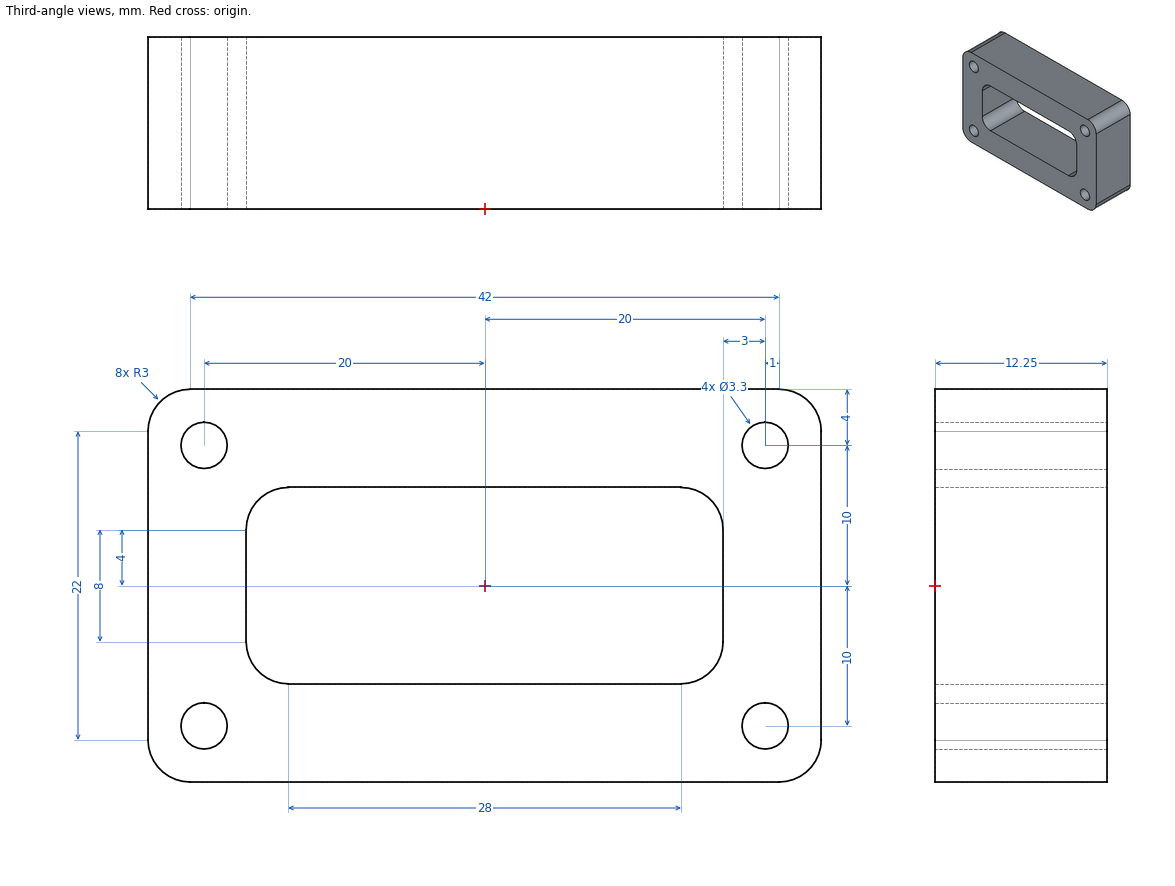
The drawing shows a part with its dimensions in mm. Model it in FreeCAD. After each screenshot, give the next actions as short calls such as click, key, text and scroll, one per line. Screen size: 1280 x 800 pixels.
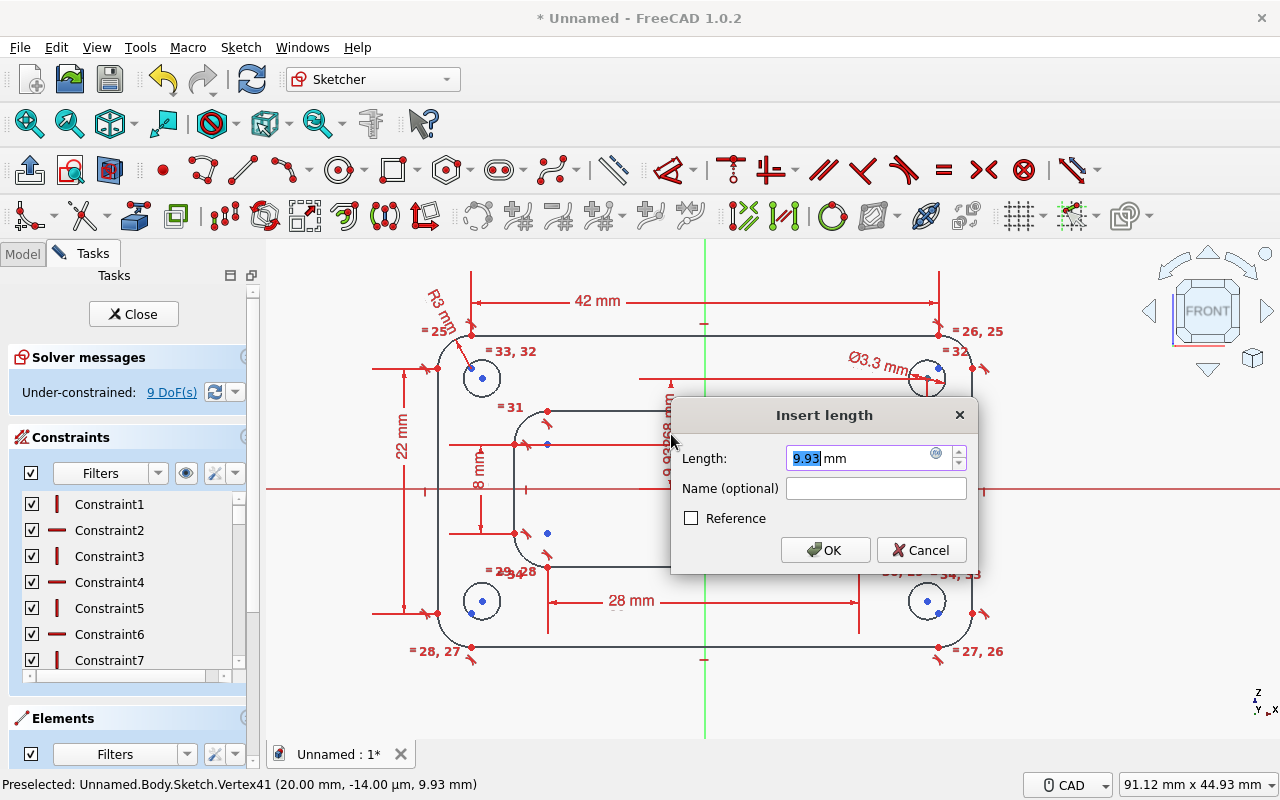
text(10)
key(Return)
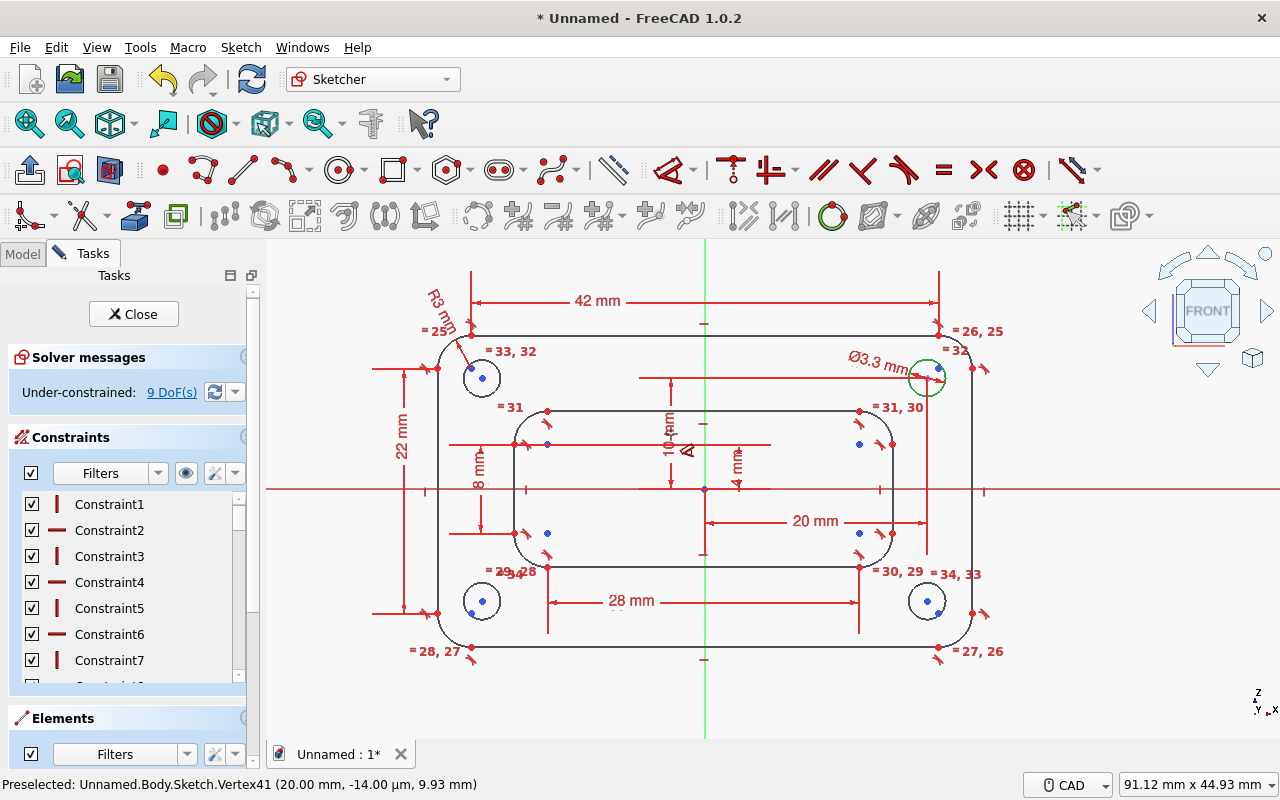
click(482, 378)
click(593, 523)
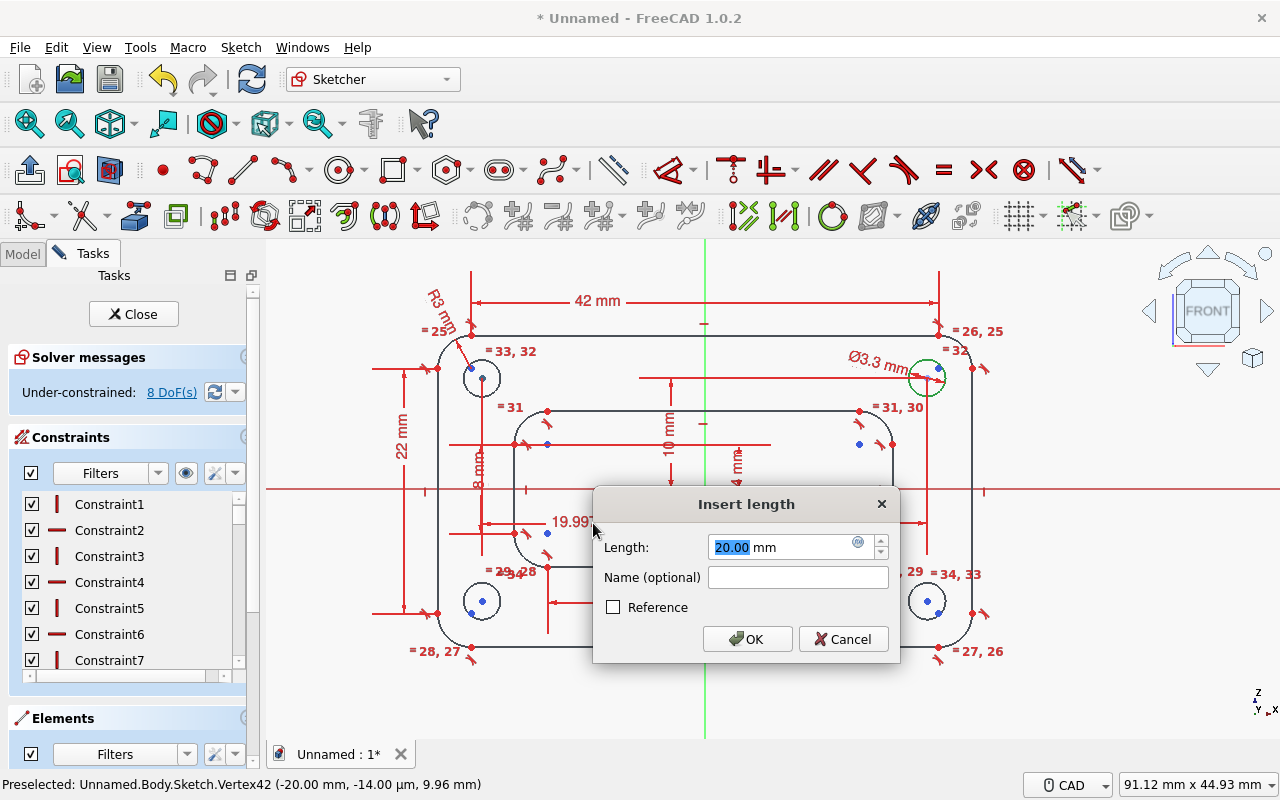
text(20)
key(Return)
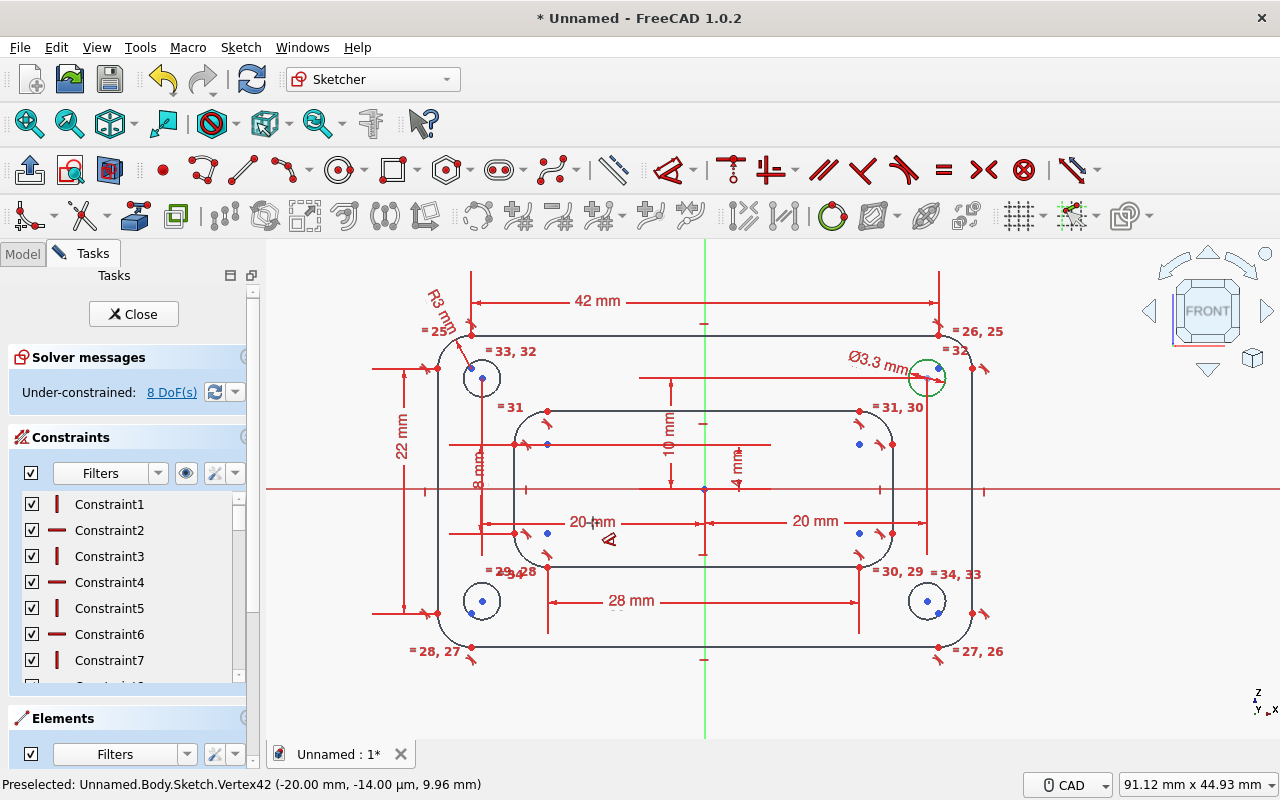
click(482, 378)
click(739, 395)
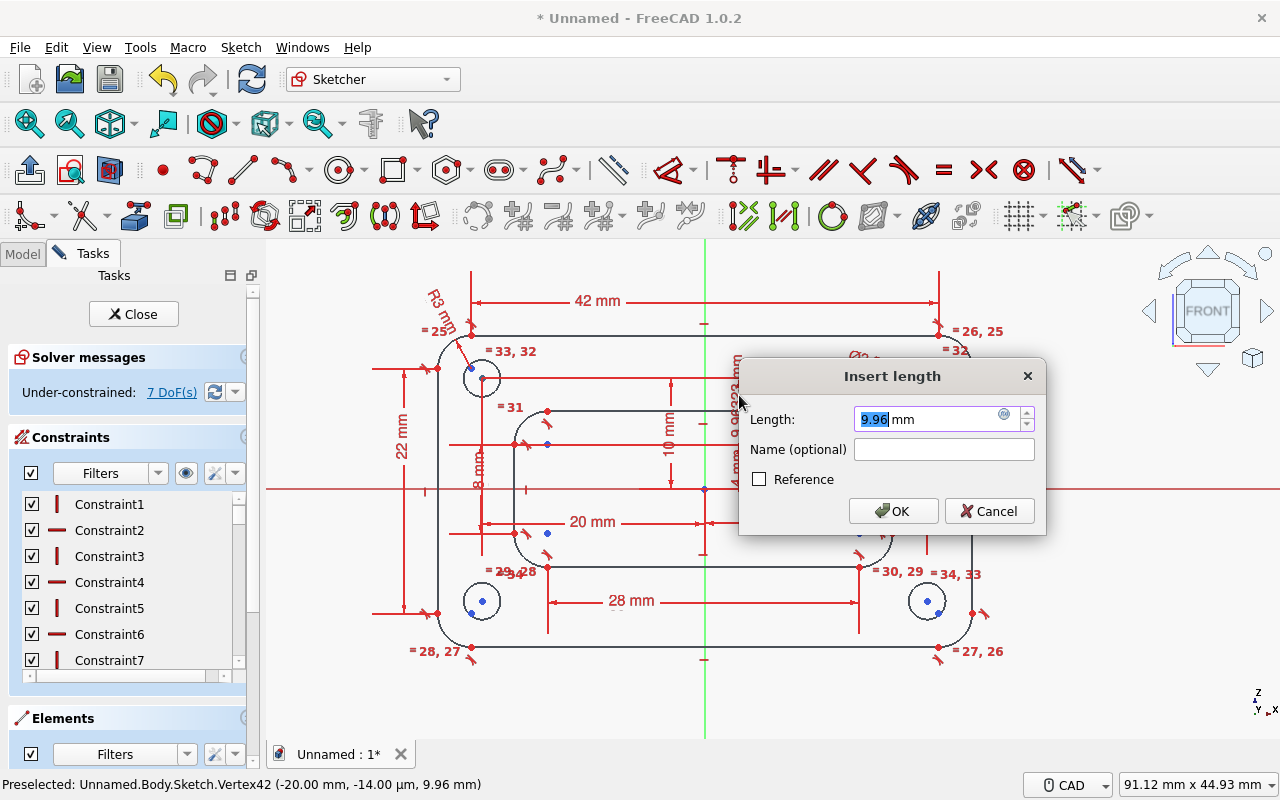
text(10)
key(Return)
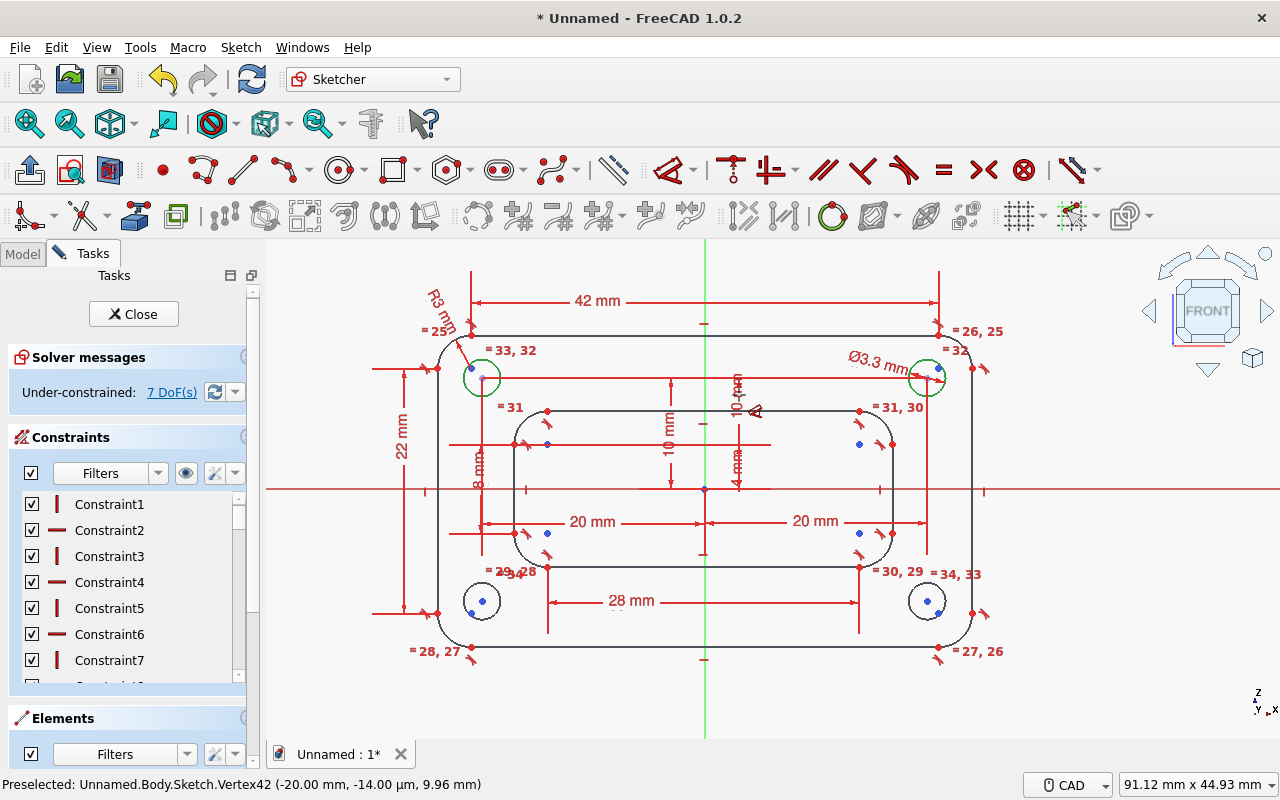
click(927, 601)
click(816, 455)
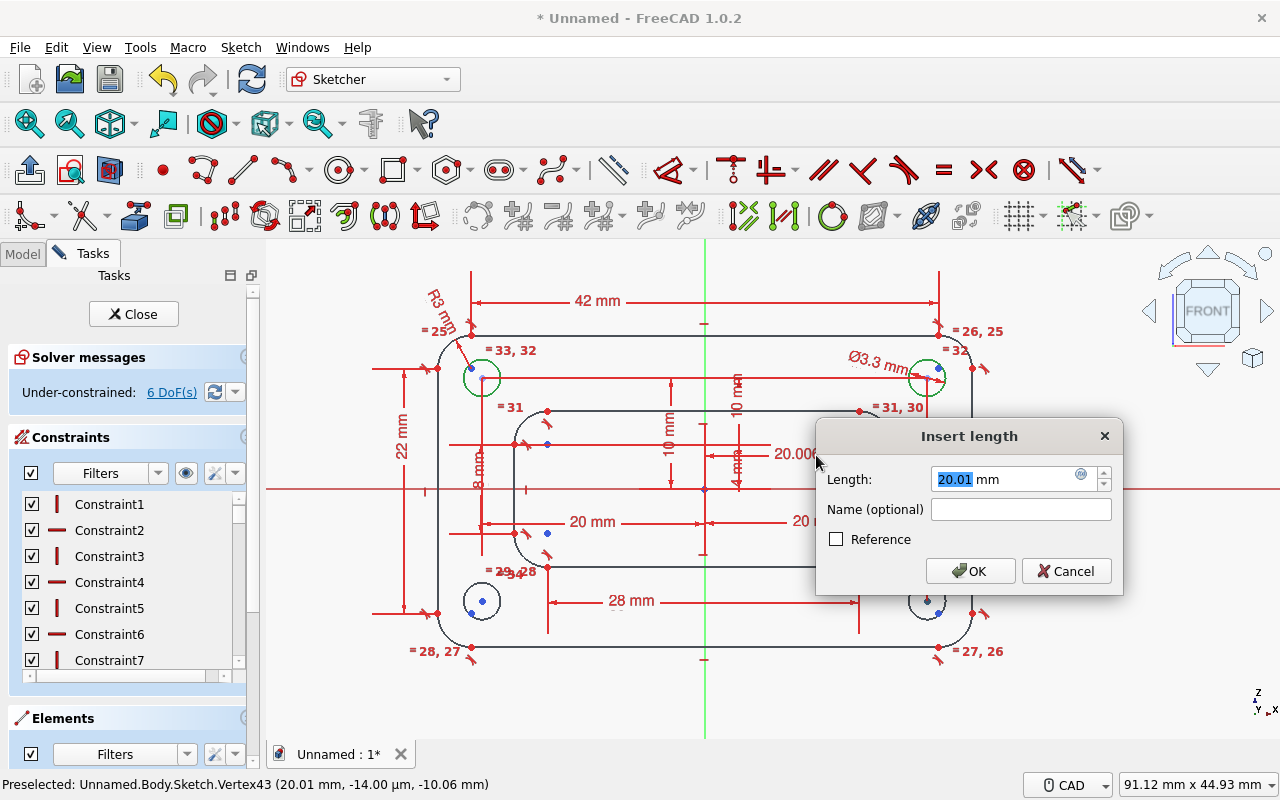
text(20)
key(Return)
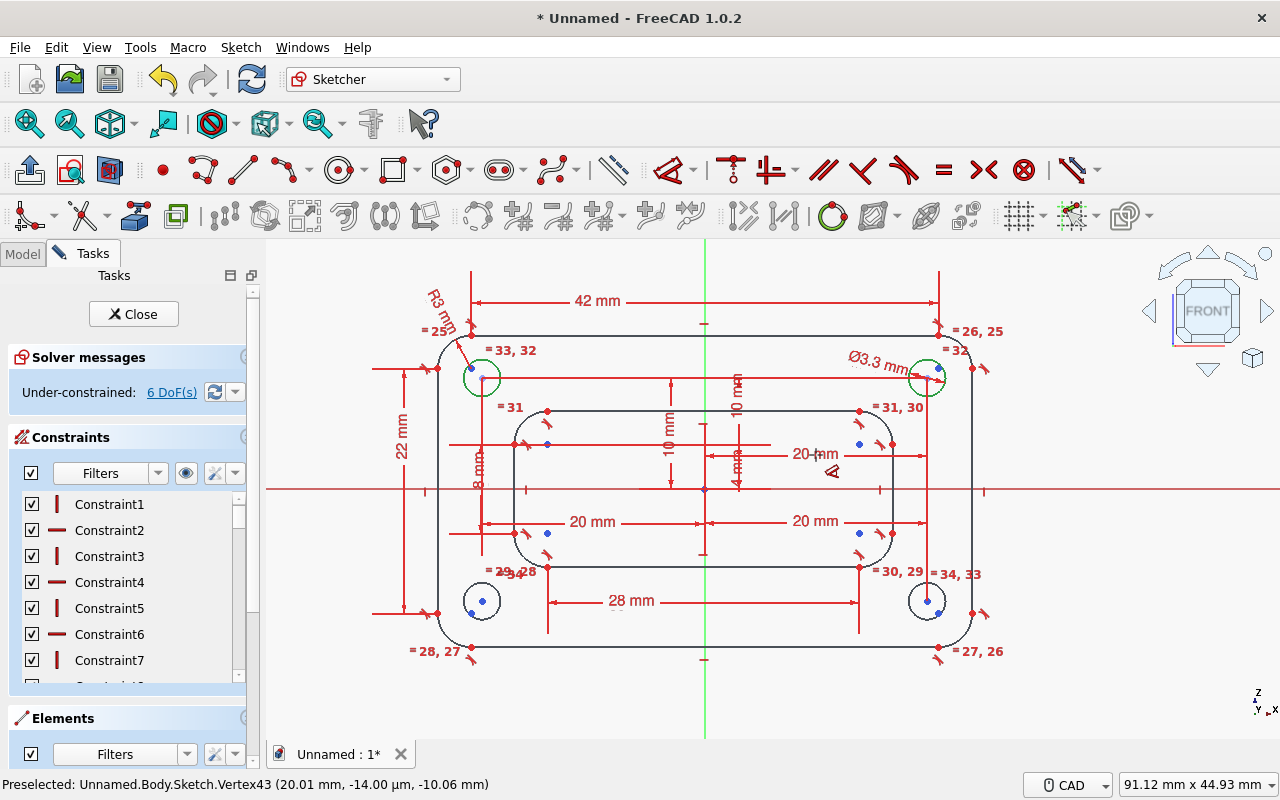
click(927, 601)
click(671, 545)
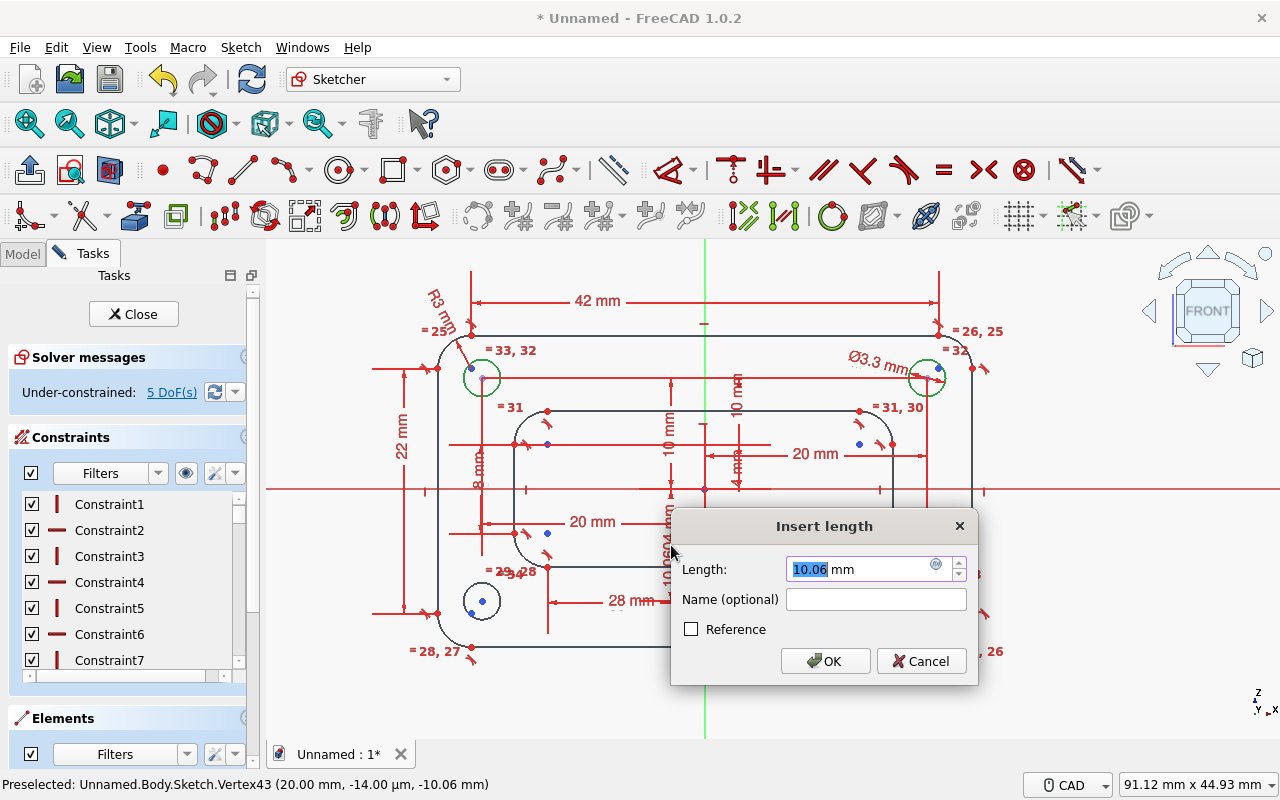
text(10)
key(Return)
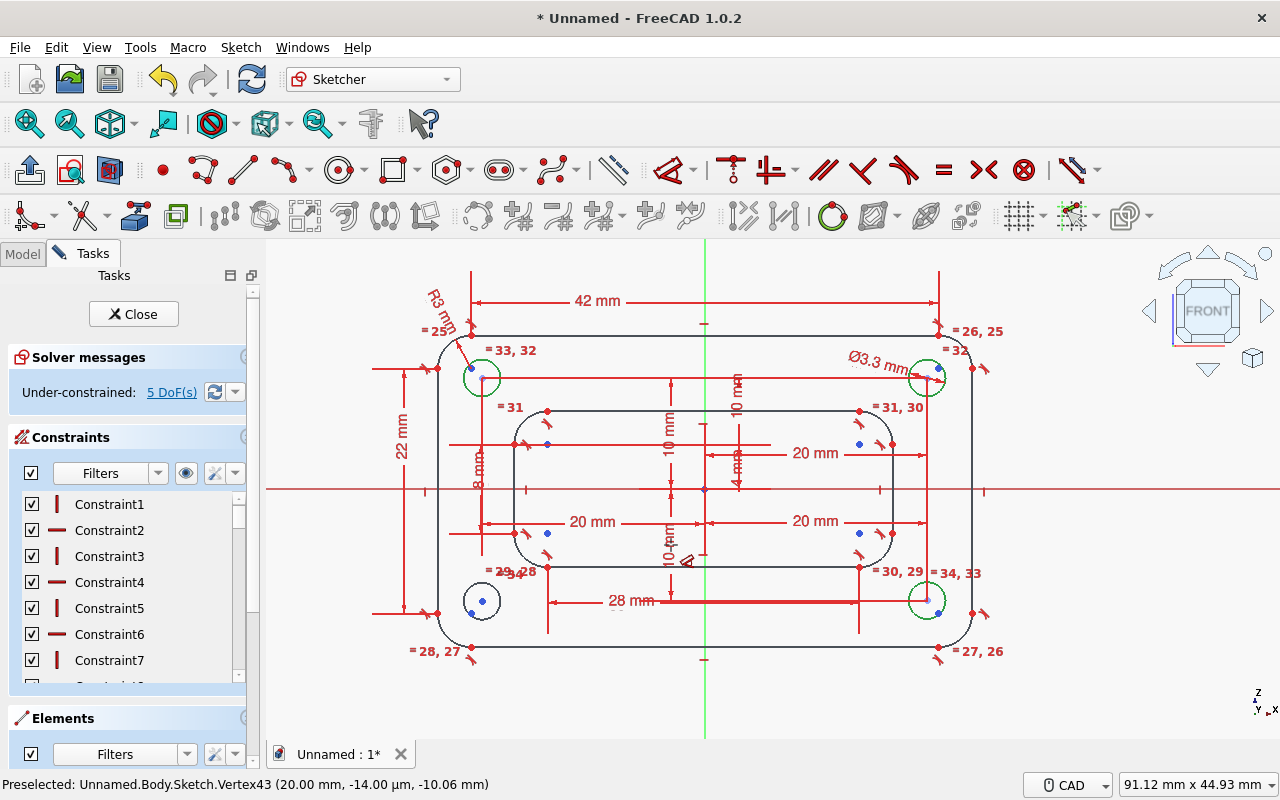
click(482, 601)
click(593, 455)